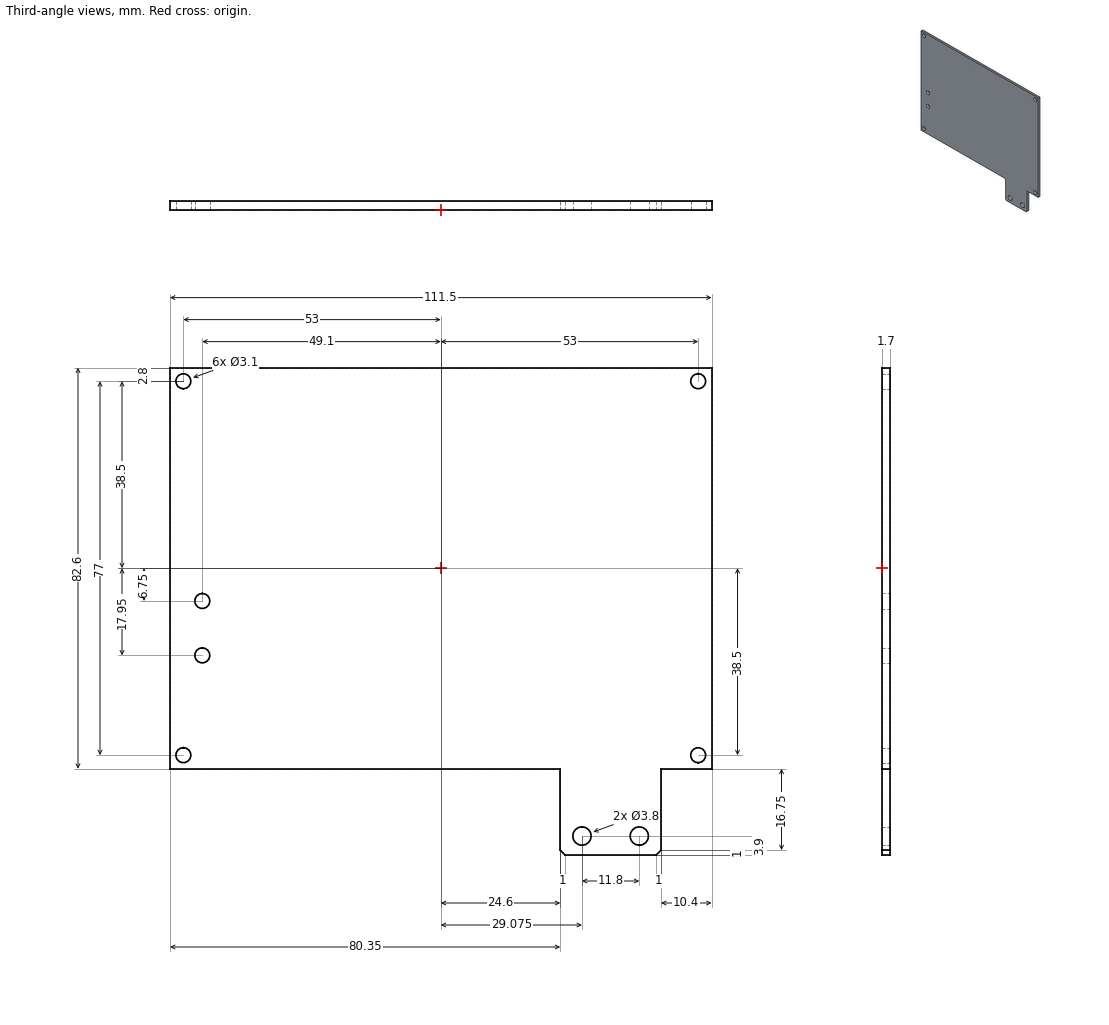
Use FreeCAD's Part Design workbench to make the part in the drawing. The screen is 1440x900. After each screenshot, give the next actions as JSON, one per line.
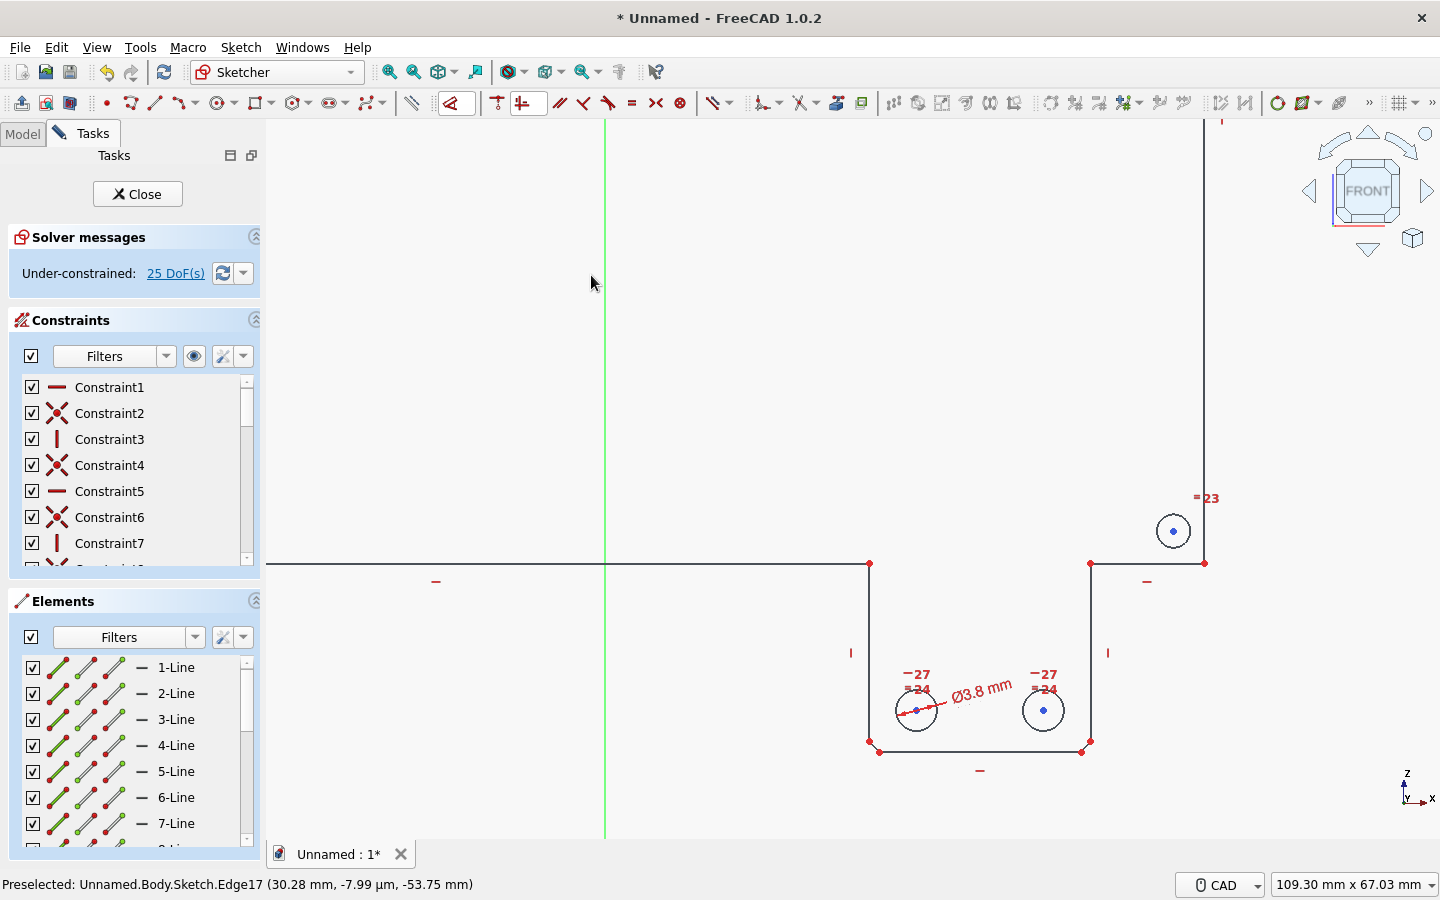
{"action": "scroll", "coordinate": [1086, 747], "scroll_direction": "up", "scroll_amount": 7}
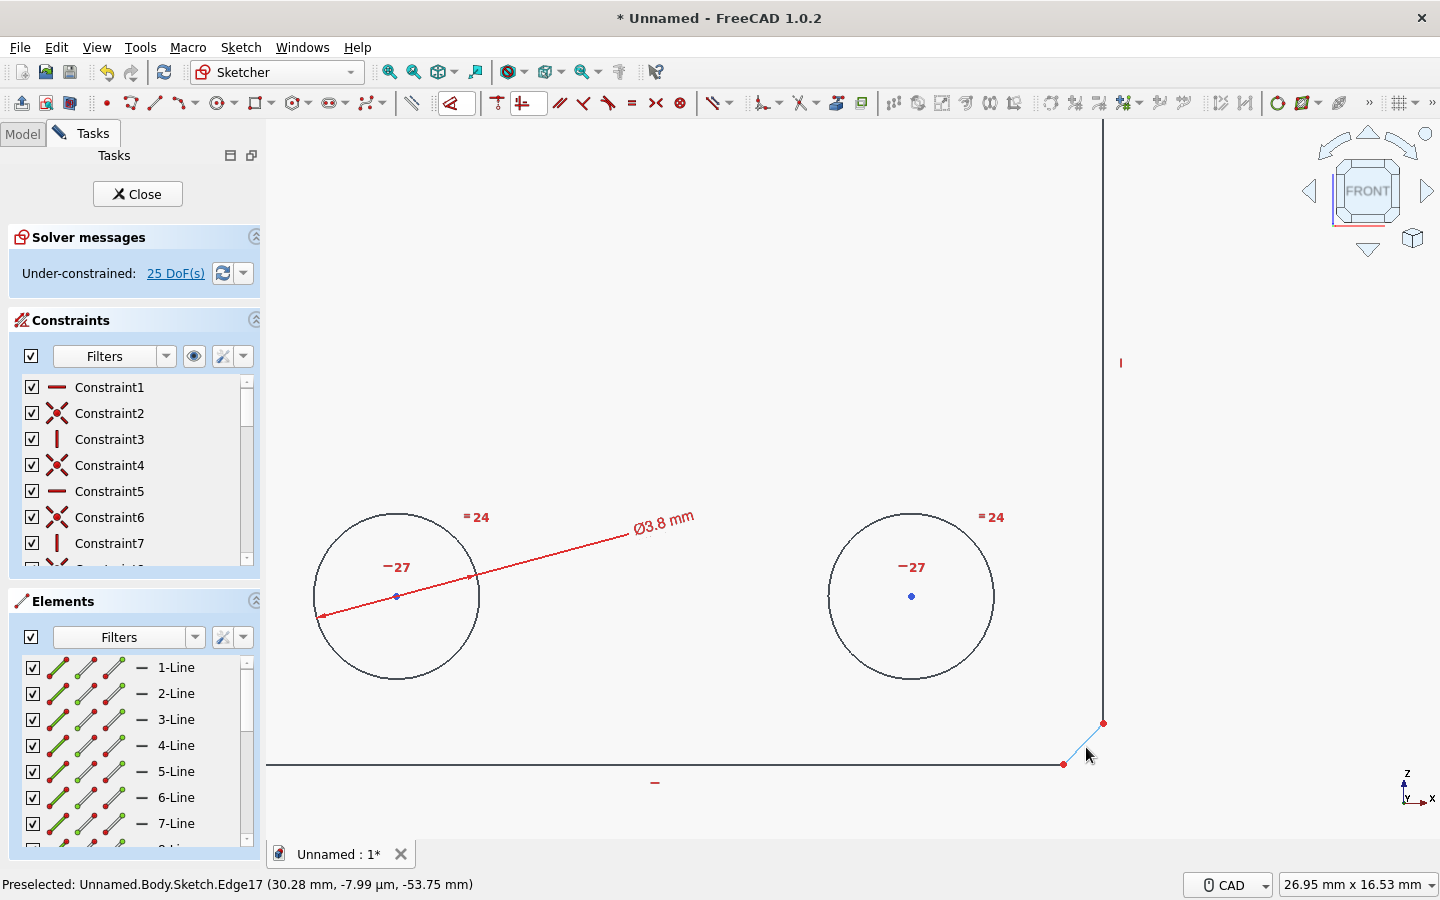
{"action": "left_click", "coordinate": [1083, 744]}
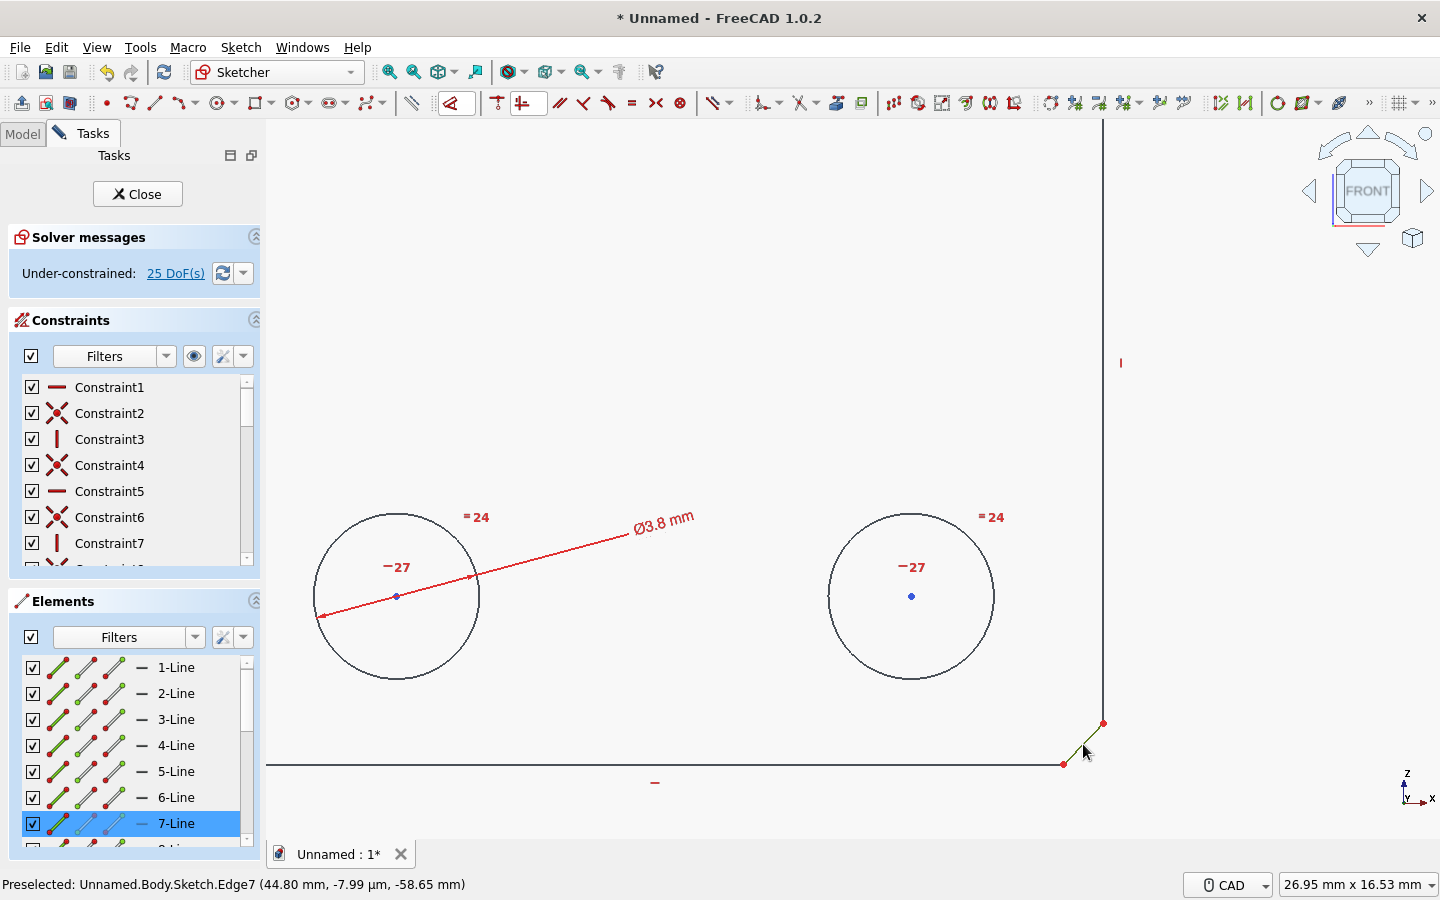
{"action": "left_click", "coordinate": [470, 104]}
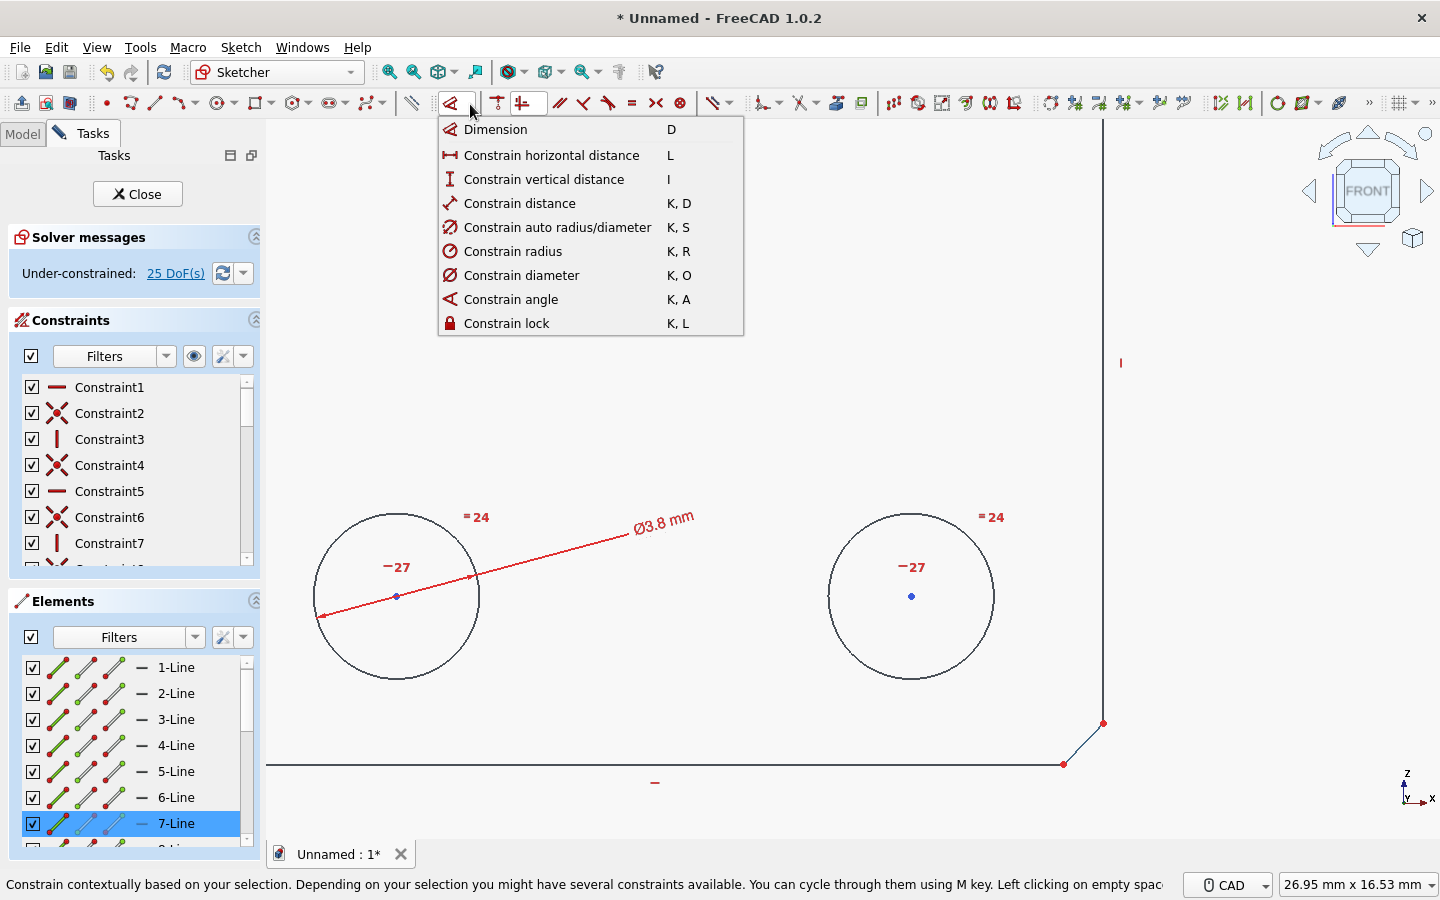
{"action": "left_click", "coordinate": [591, 155]}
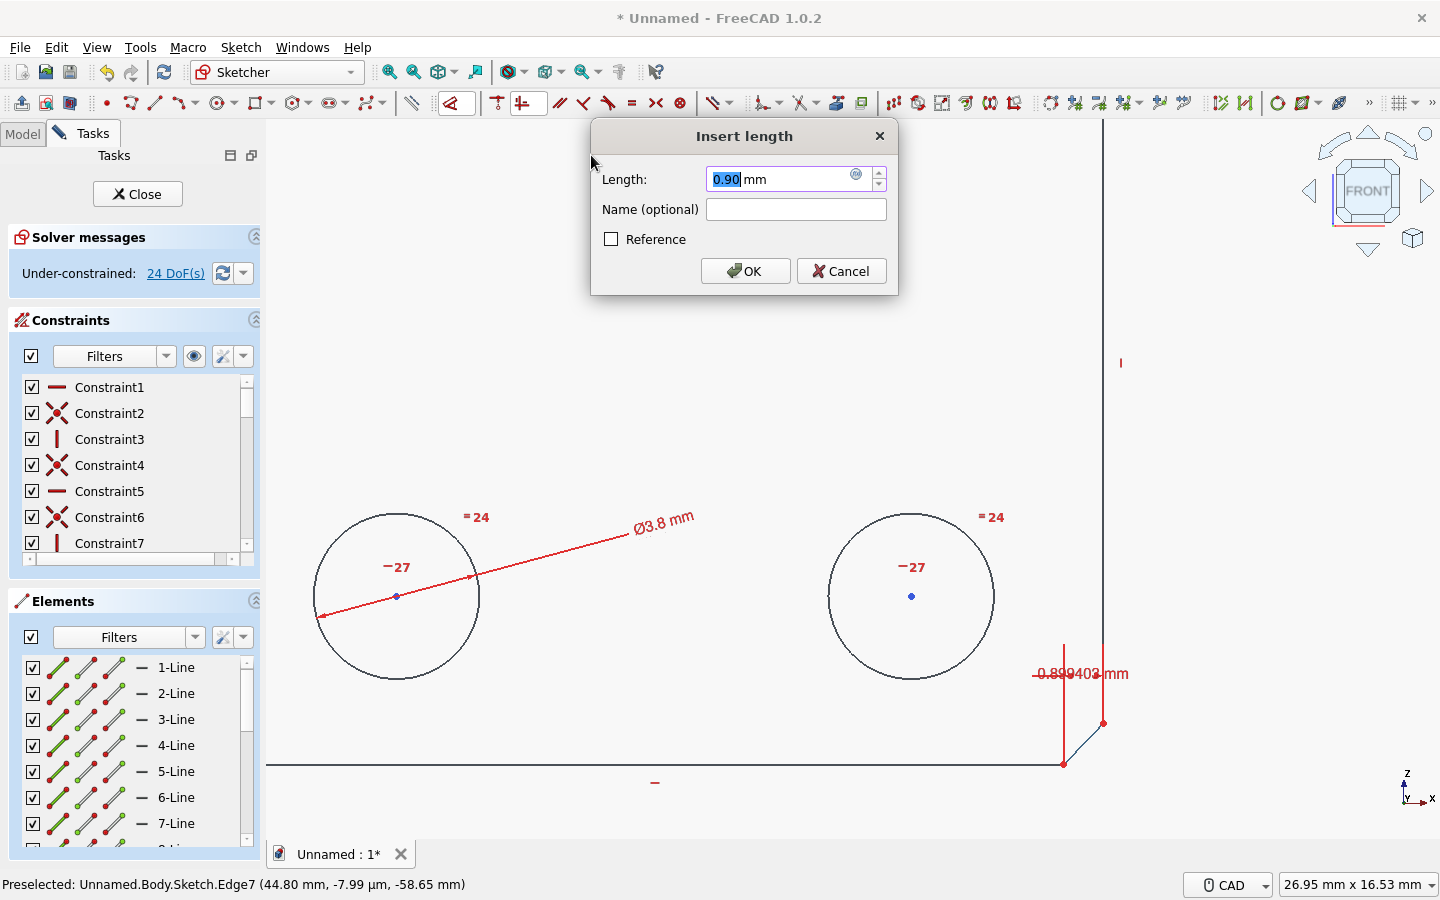
{"action": "type", "text": "1"}
{"action": "key", "text": "Return"}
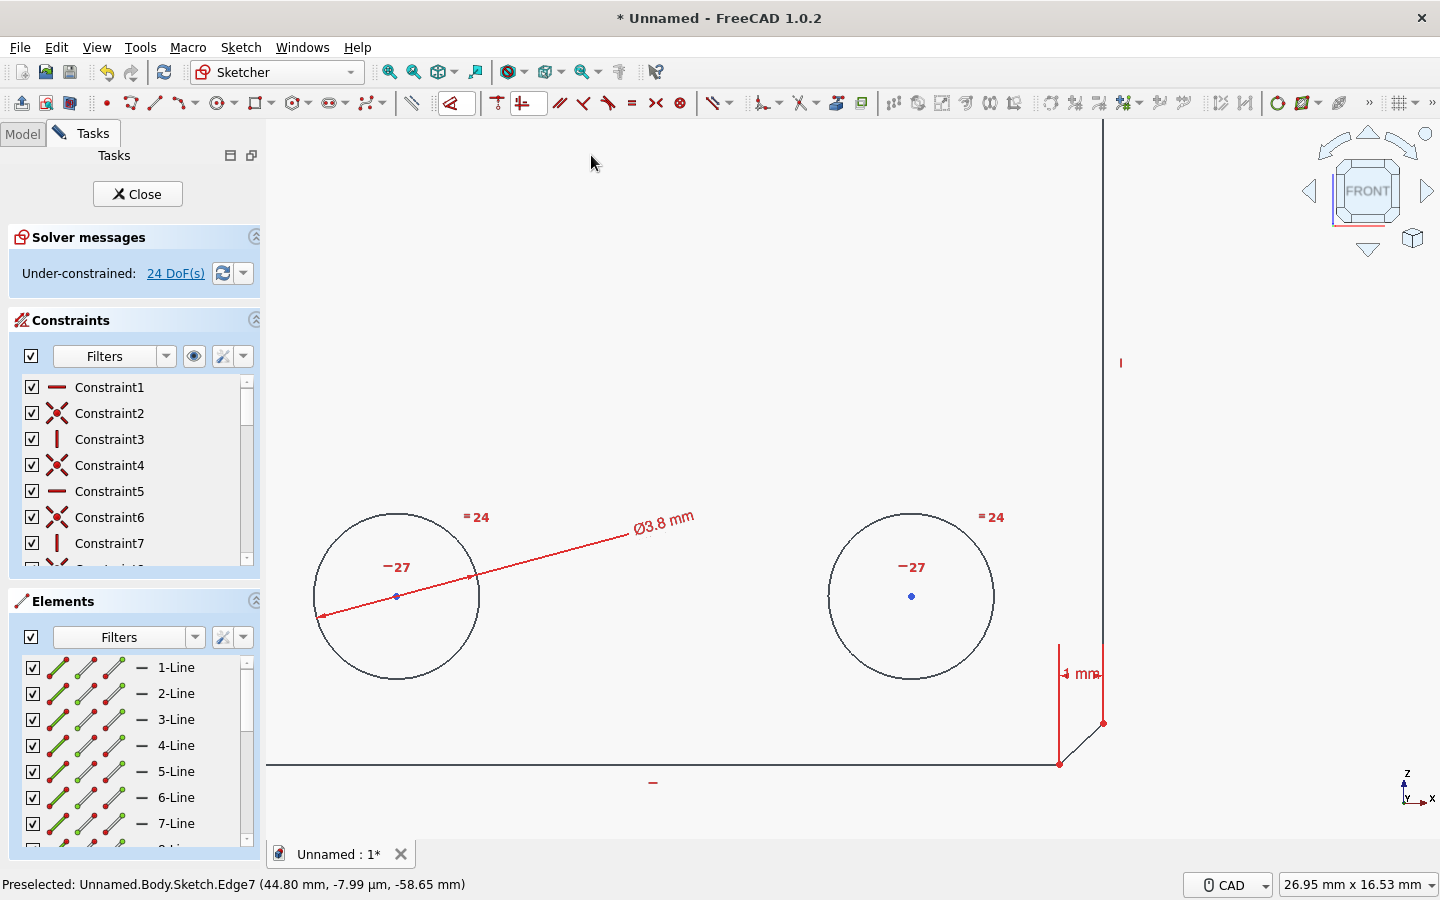
{"action": "left_click", "coordinate": [1090, 736]}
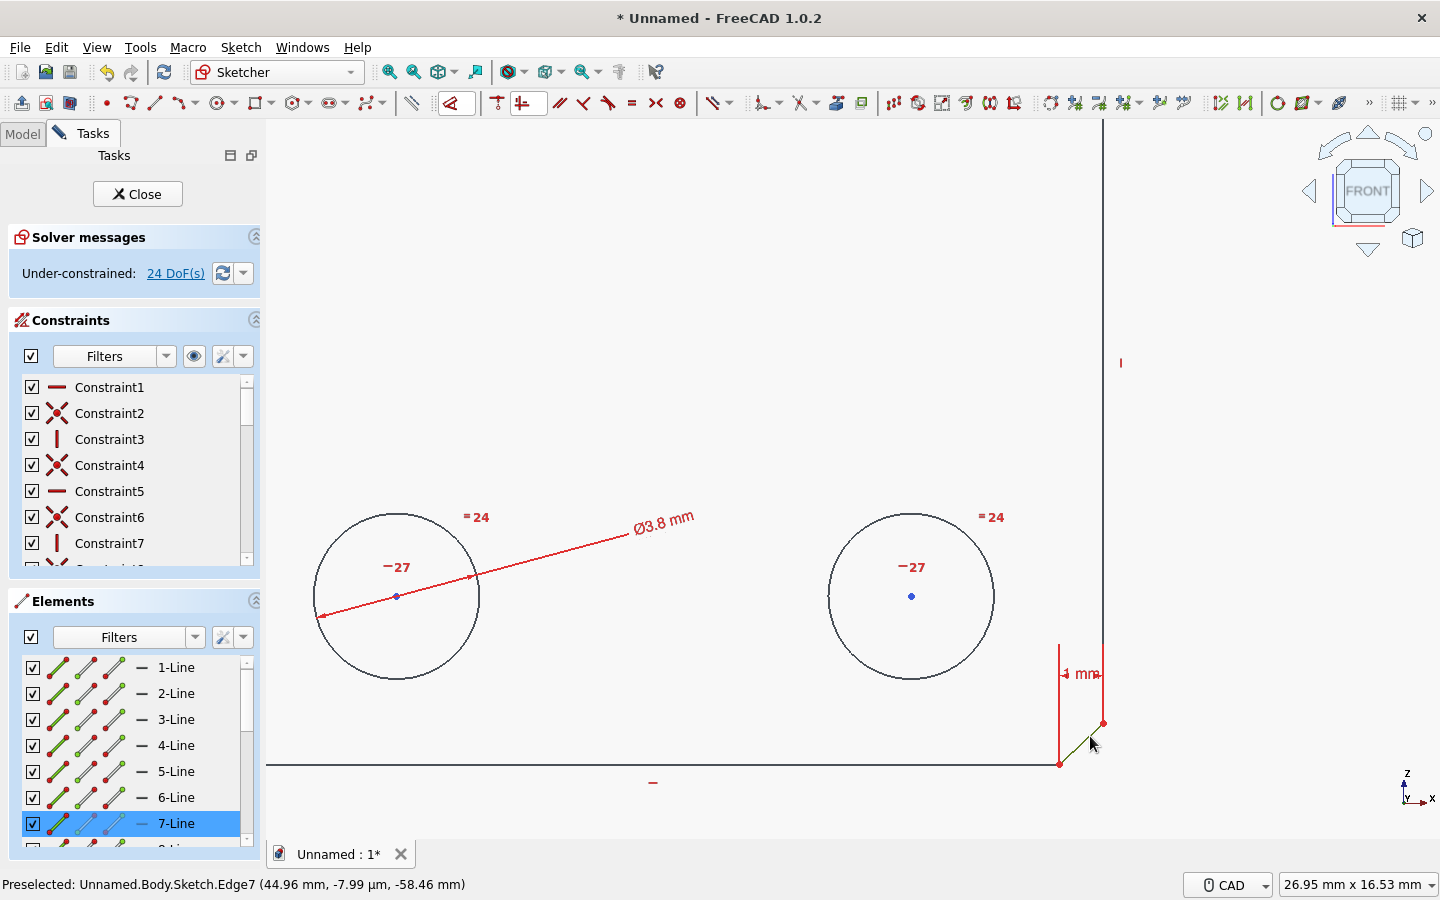
{"action": "left_click", "coordinate": [470, 104]}